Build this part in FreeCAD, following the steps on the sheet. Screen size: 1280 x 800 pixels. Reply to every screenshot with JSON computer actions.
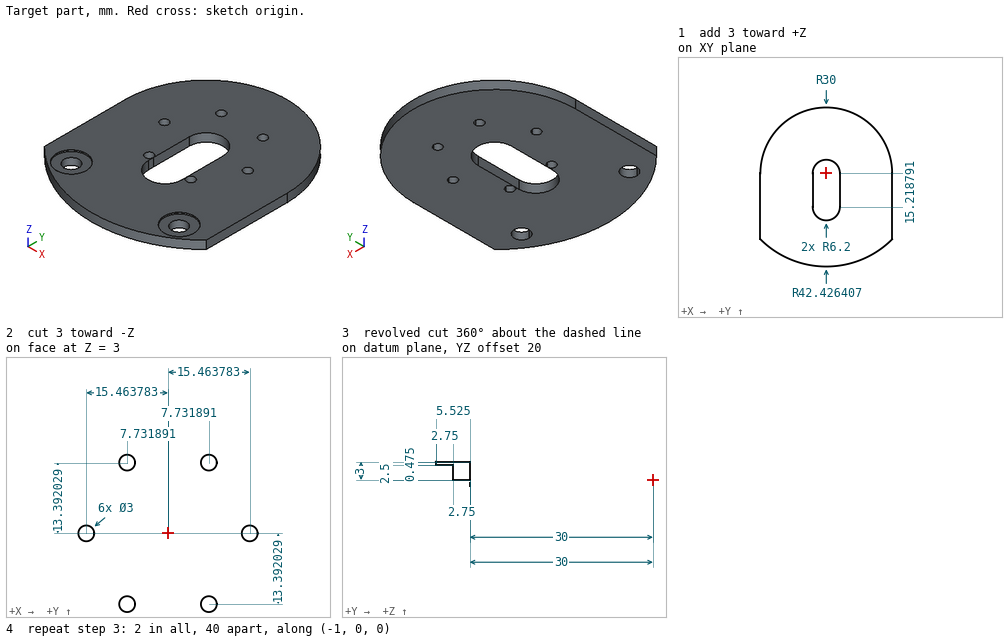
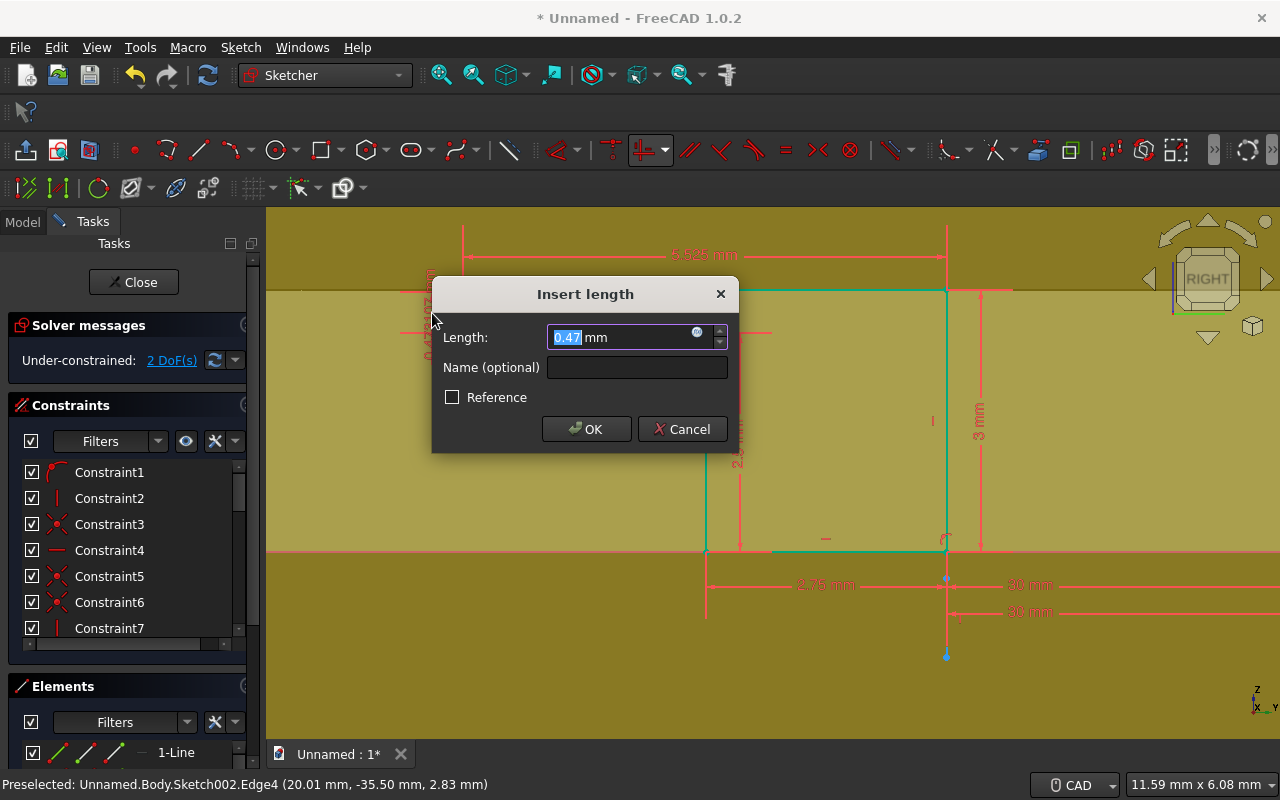
{"action": "type", "text": "0.475"}
{"action": "key", "text": "Return"}
{"action": "key", "text": "Escape"}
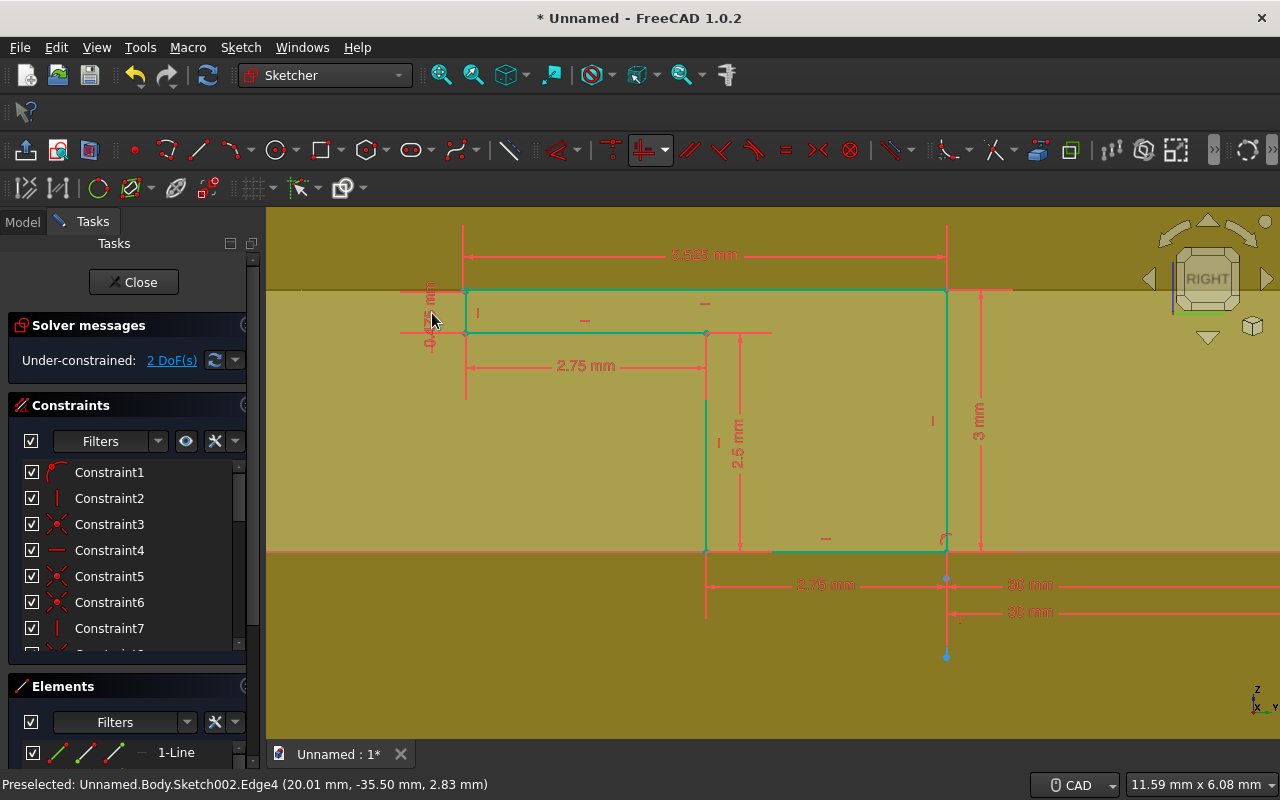
{"action": "left_click", "coordinate": [134, 282]}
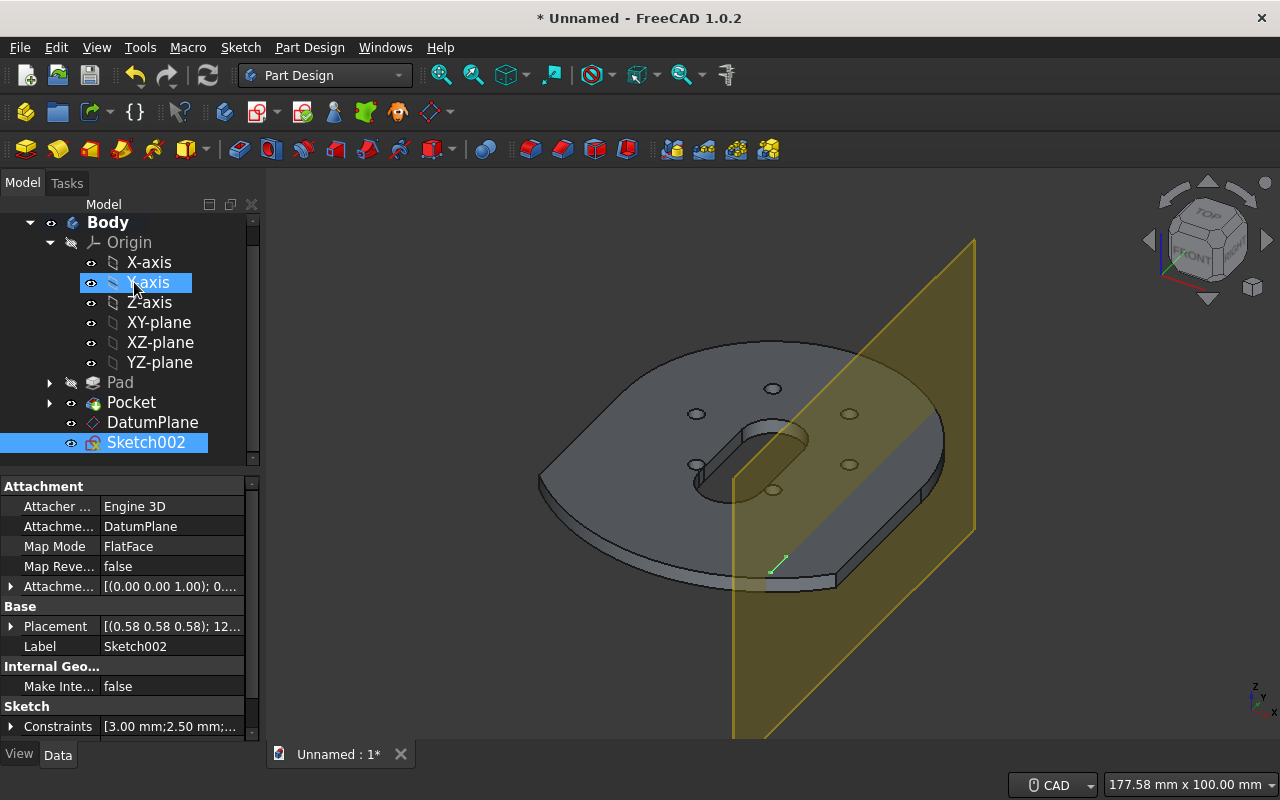
{"action": "left_click", "coordinate": [304, 150]}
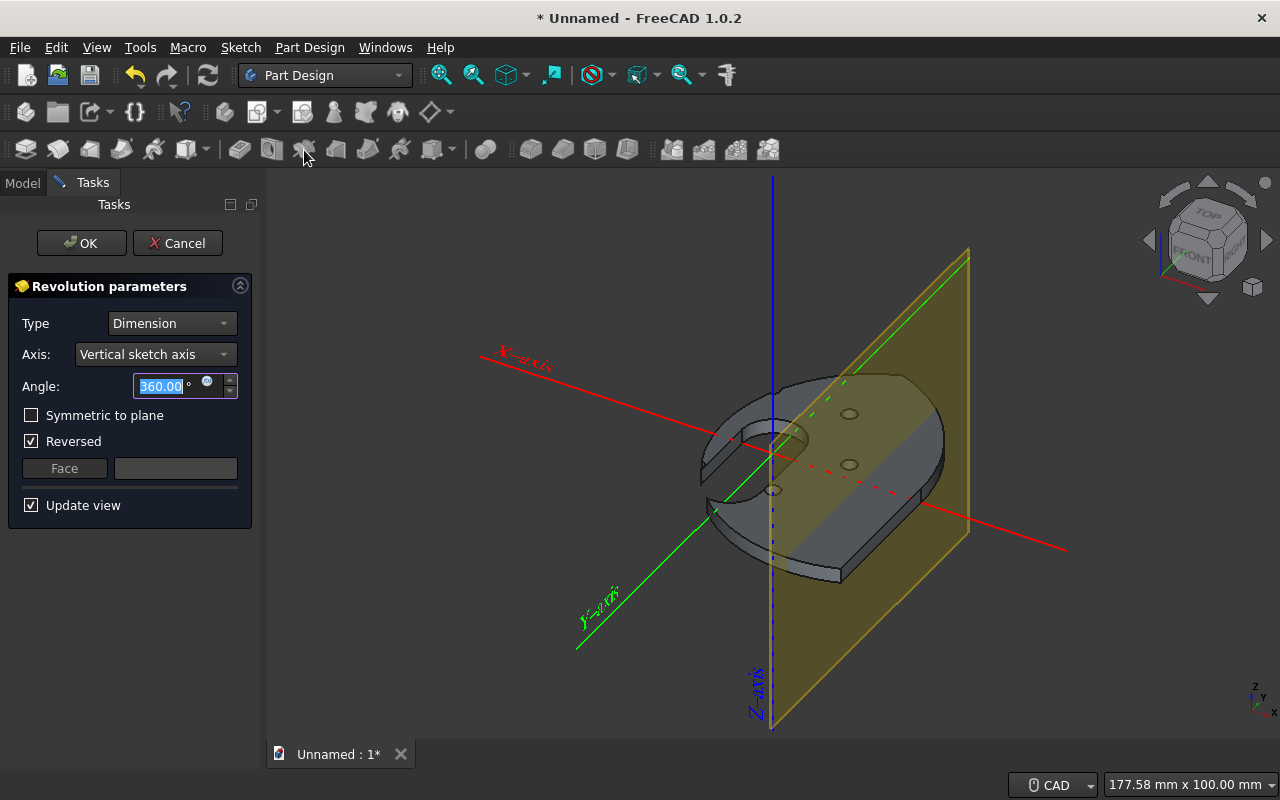
{"action": "left_click", "coordinate": [156, 354]}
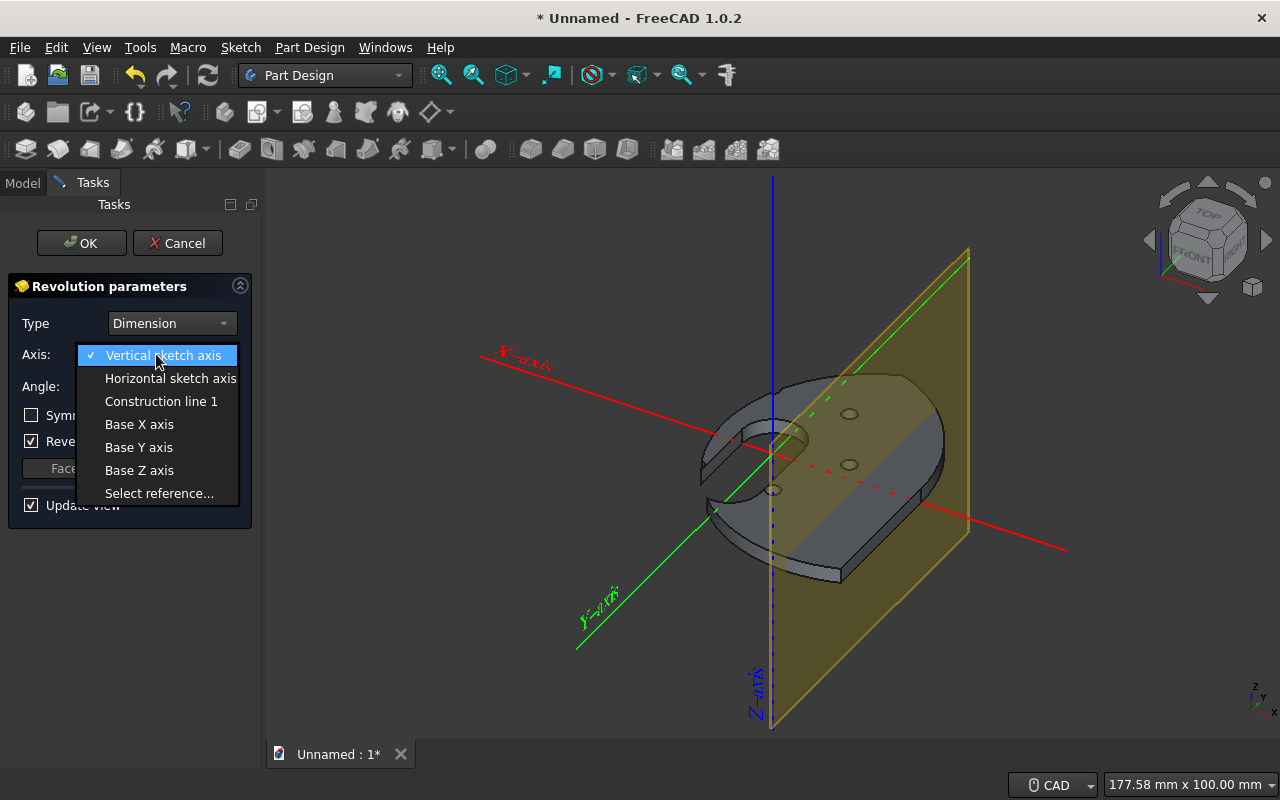
{"action": "left_click", "coordinate": [156, 402]}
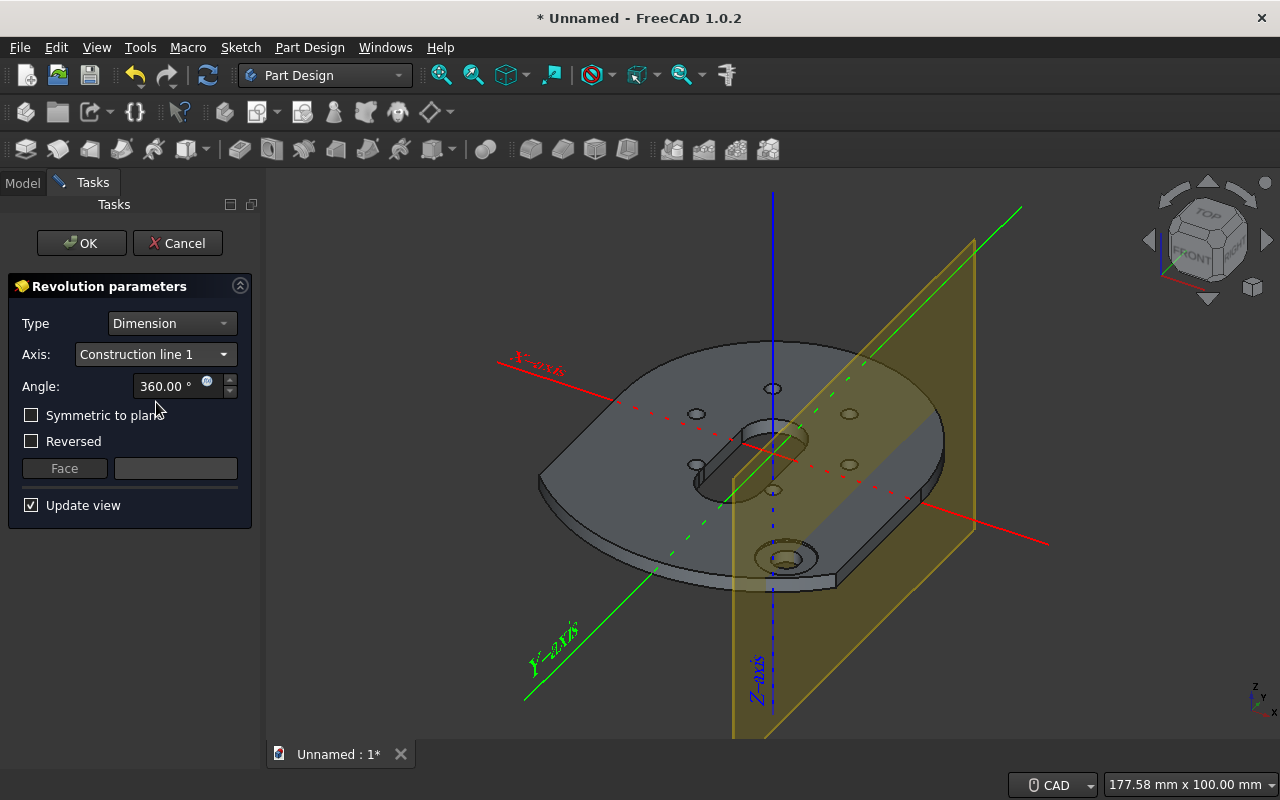
{"action": "left_click", "coordinate": [82, 243]}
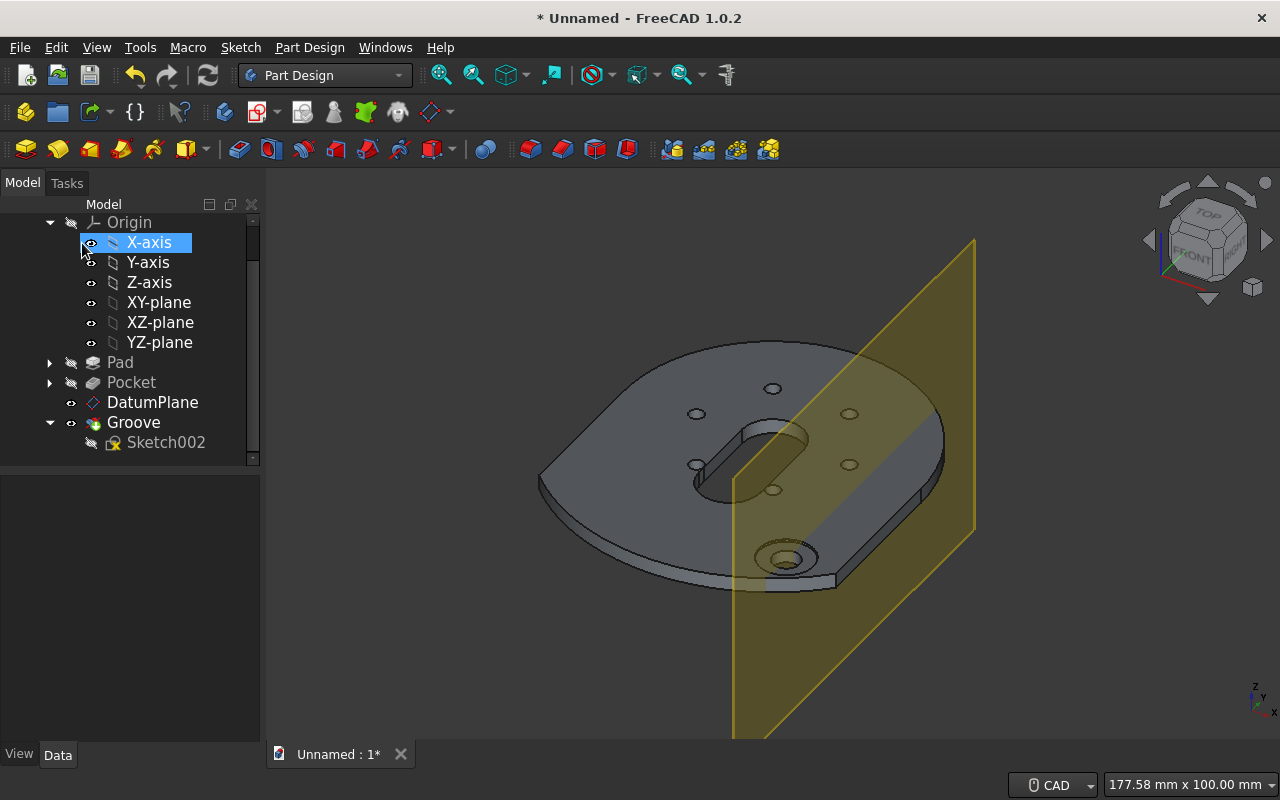
{"action": "left_click", "coordinate": [116, 403]}
{"action": "key", "text": "space"}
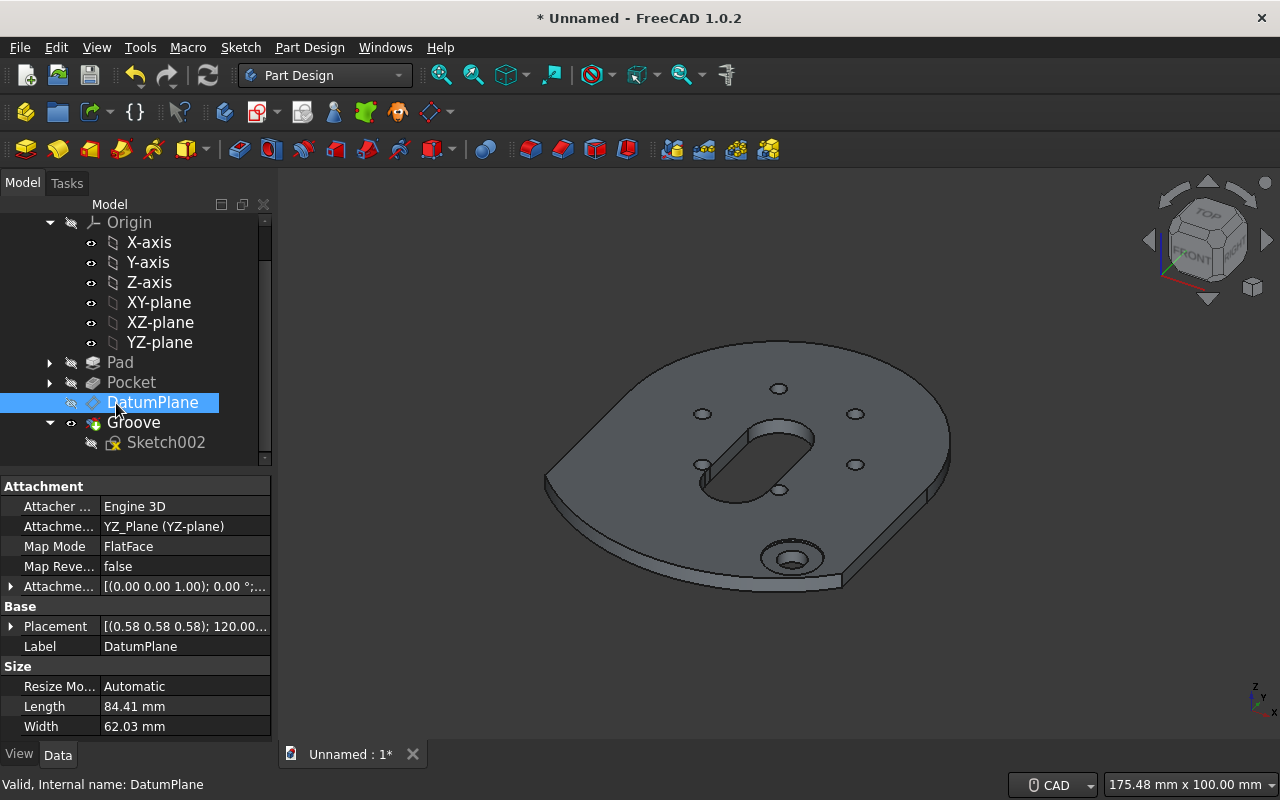
{"action": "left_click", "coordinate": [116, 423]}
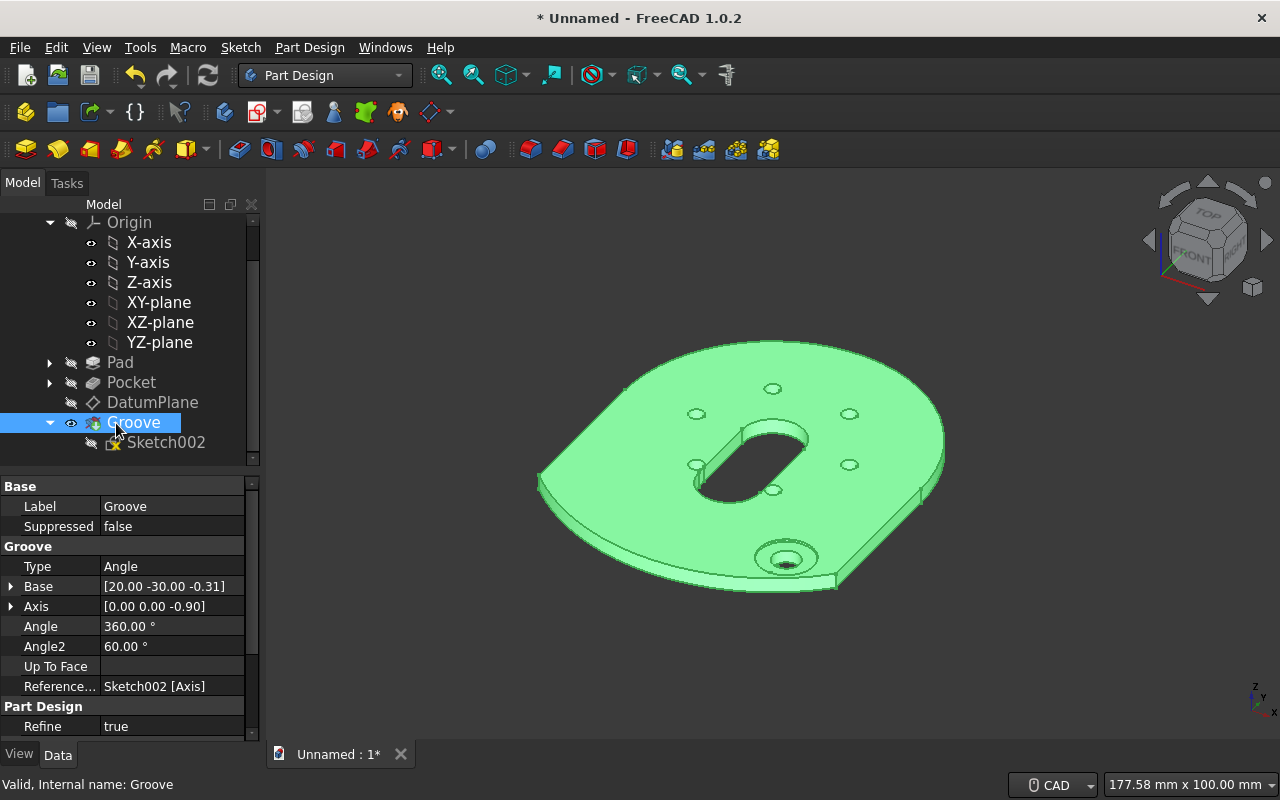
{"action": "left_click", "coordinate": [704, 150]}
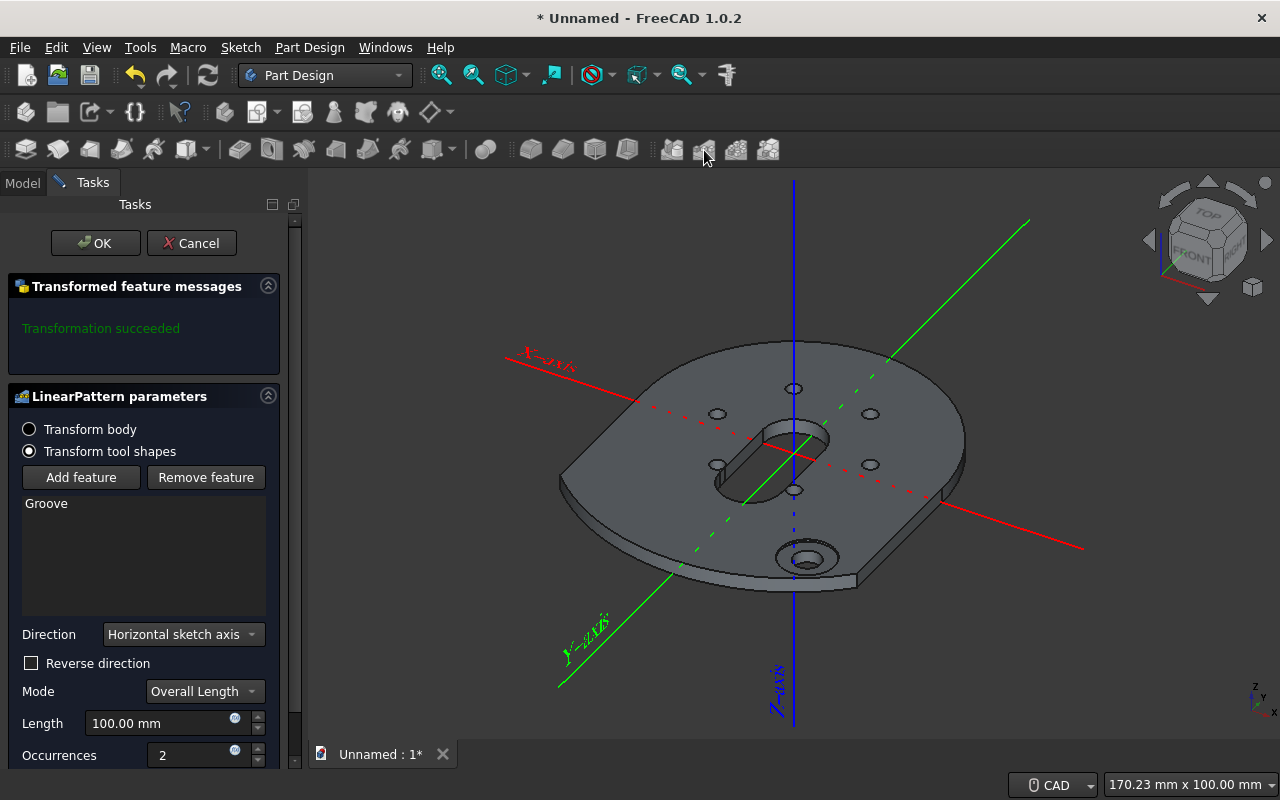
{"action": "left_click", "coordinate": [184, 634]}